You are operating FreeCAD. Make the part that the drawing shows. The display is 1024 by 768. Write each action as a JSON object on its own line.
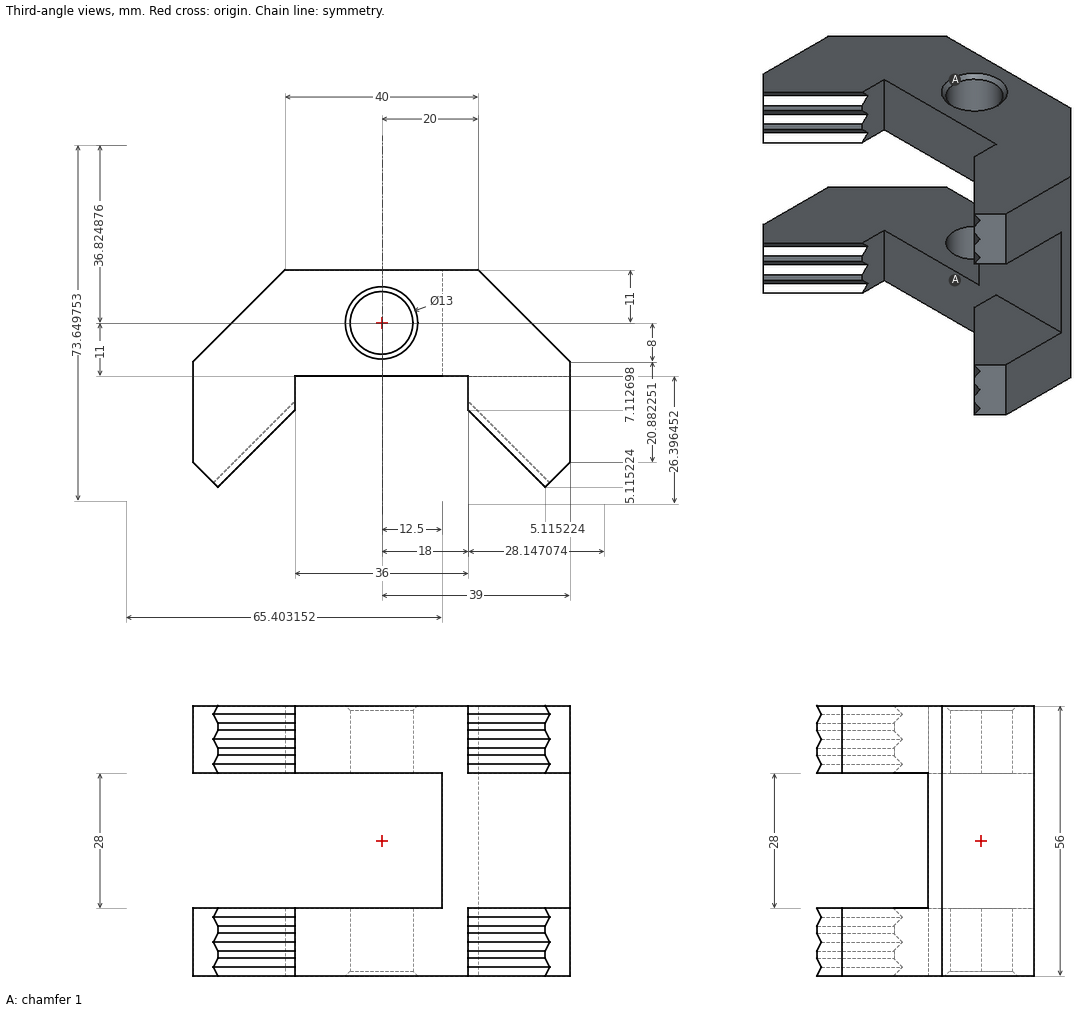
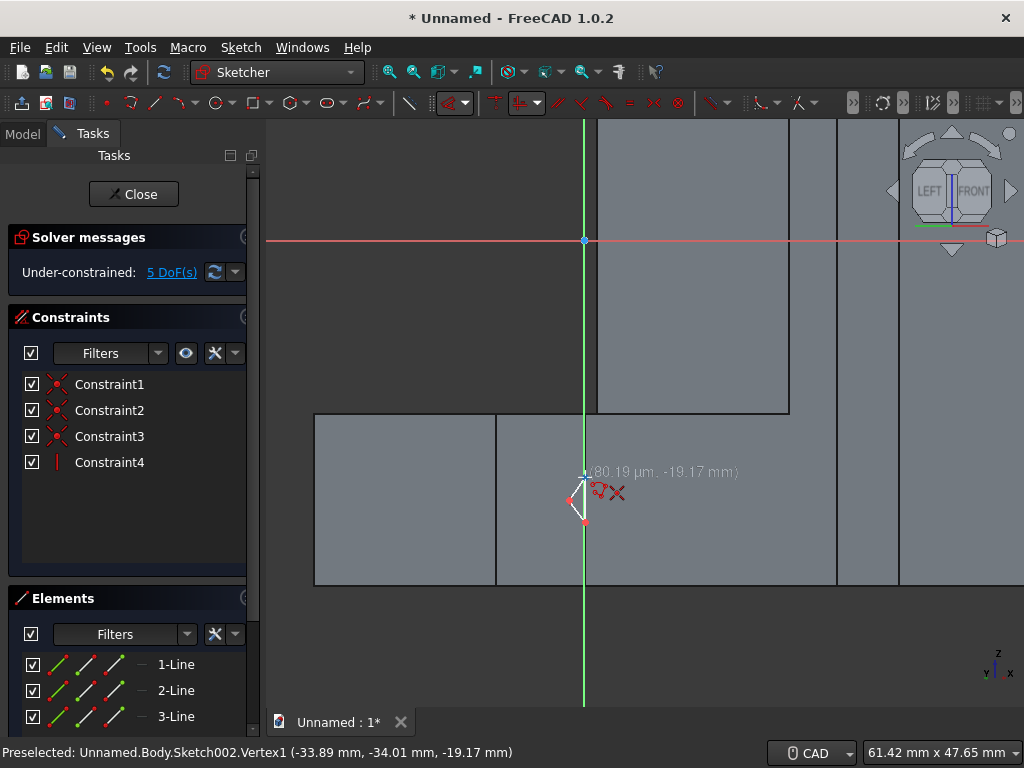
{"action": "scroll", "coordinate": [585, 414], "scroll_direction": "up", "scroll_amount": 14}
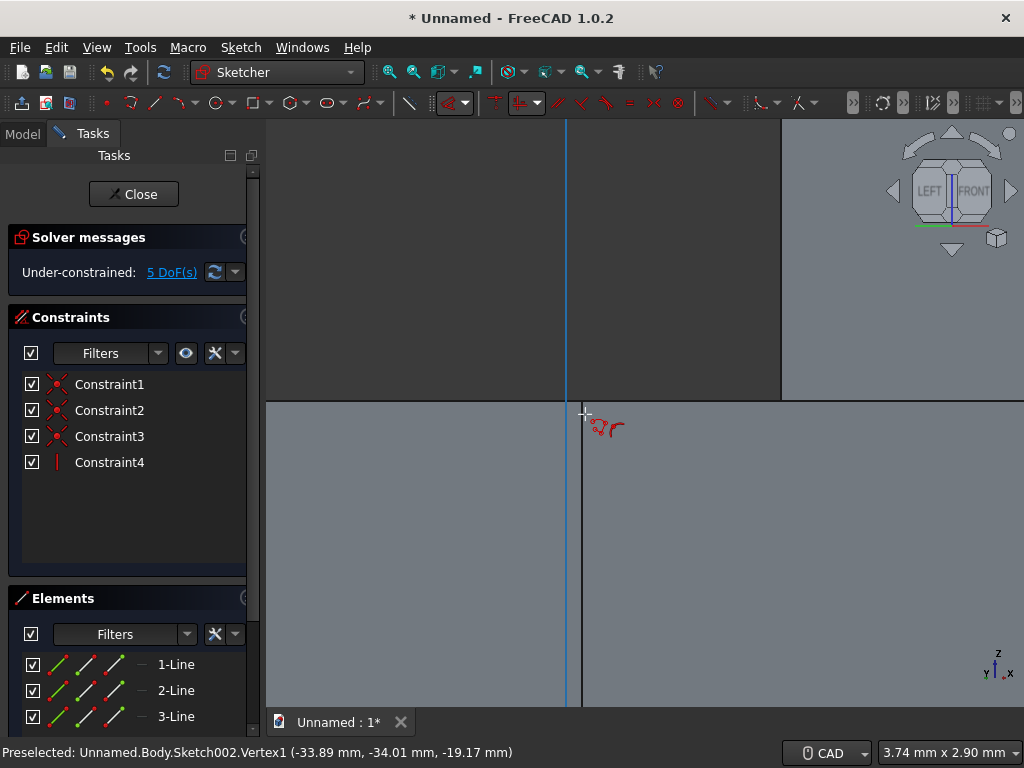
{"action": "left_click", "coordinate": [582, 401]}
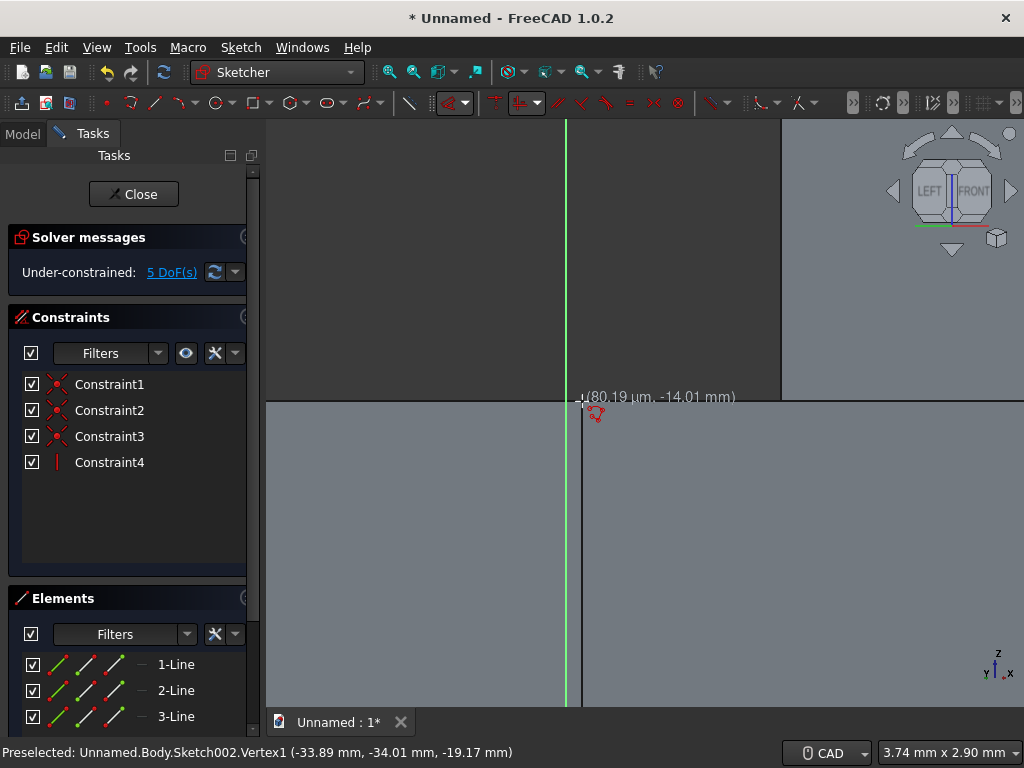
{"action": "scroll", "coordinate": [585, 414], "scroll_direction": "down", "scroll_amount": 14}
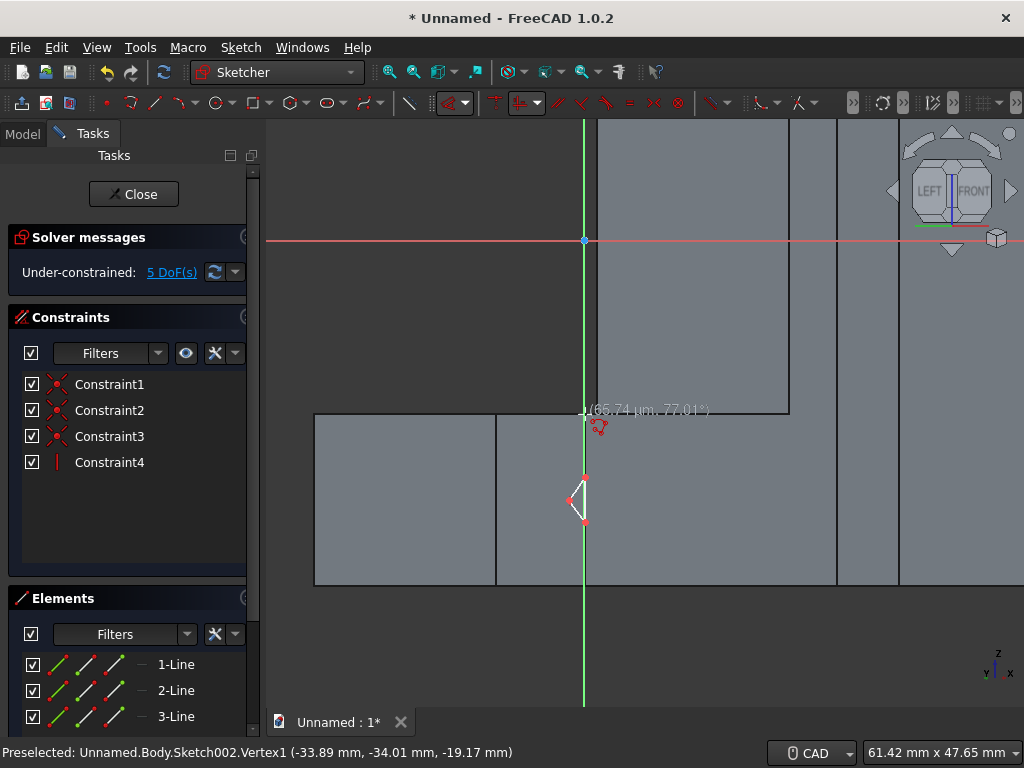
{"action": "left_click", "coordinate": [569, 436]}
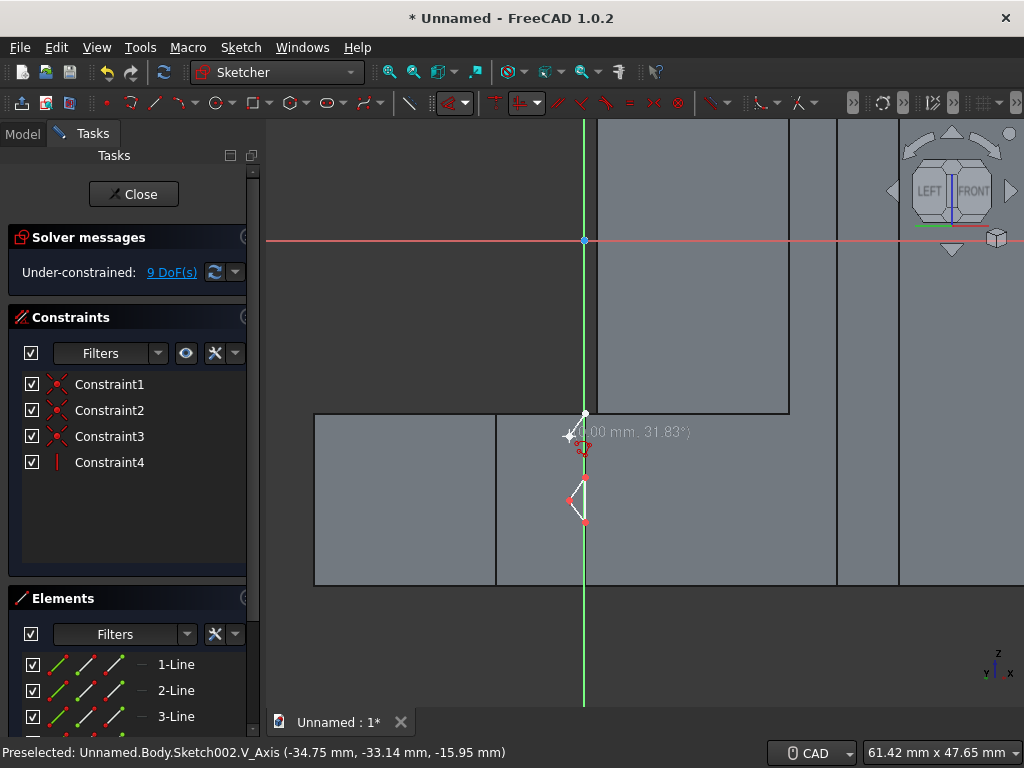
{"action": "scroll", "coordinate": [585, 459], "scroll_direction": "up", "scroll_amount": 14}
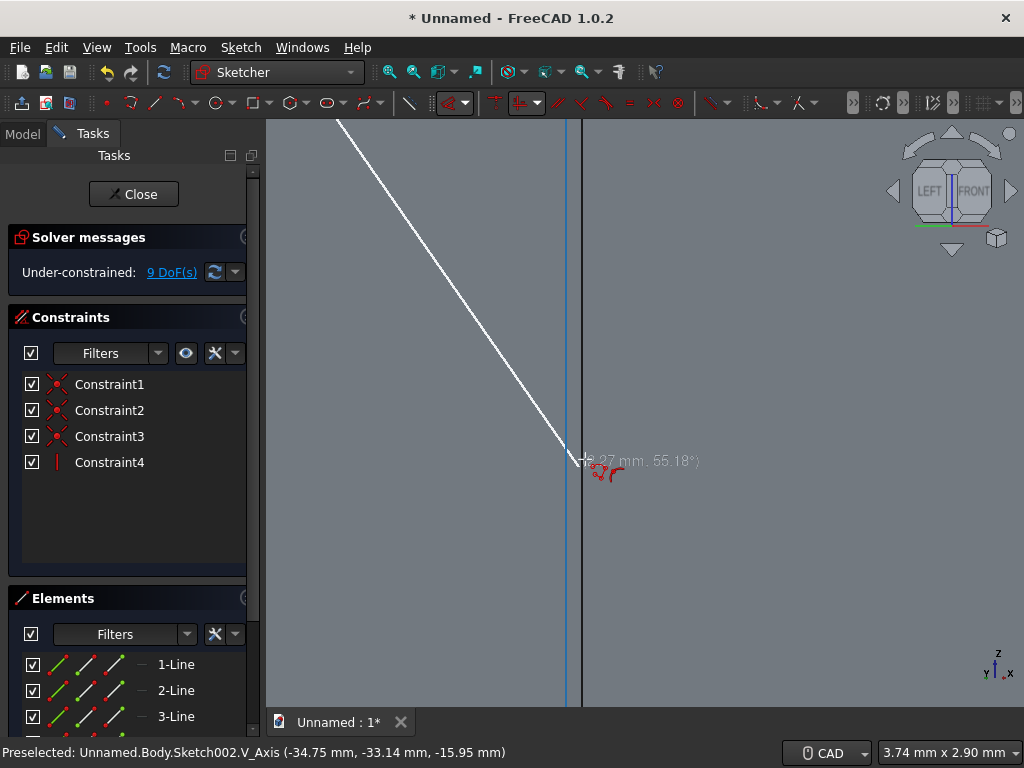
{"action": "left_click", "coordinate": [582, 449]}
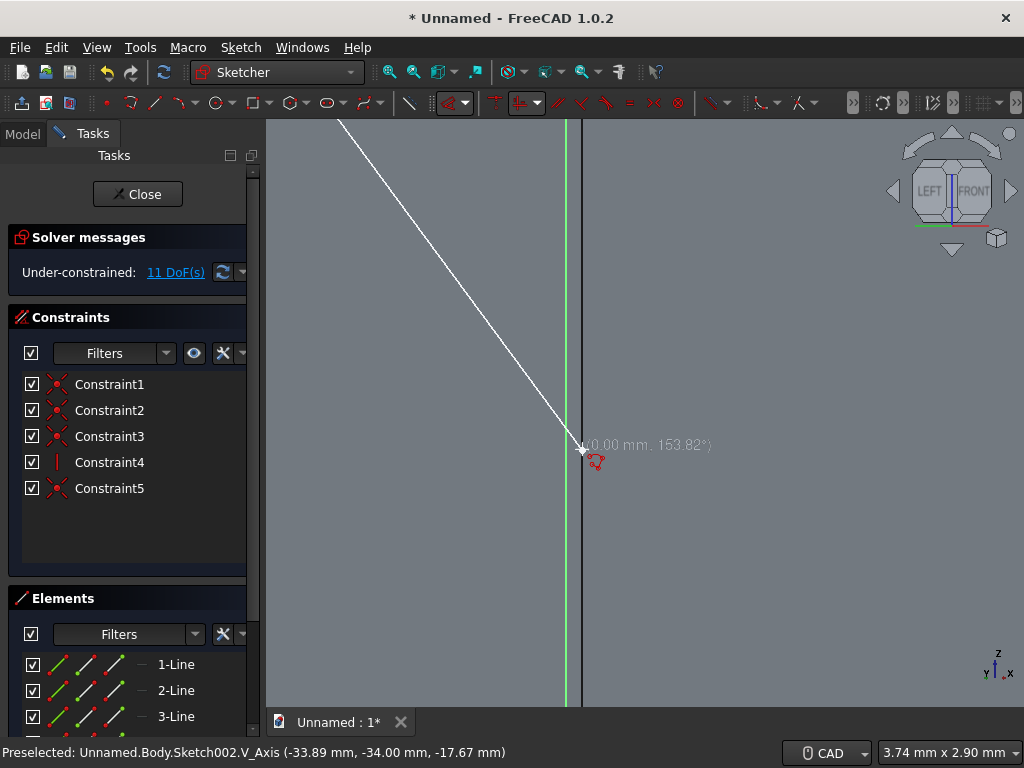
{"action": "scroll", "coordinate": [585, 459], "scroll_direction": "down", "scroll_amount": 14}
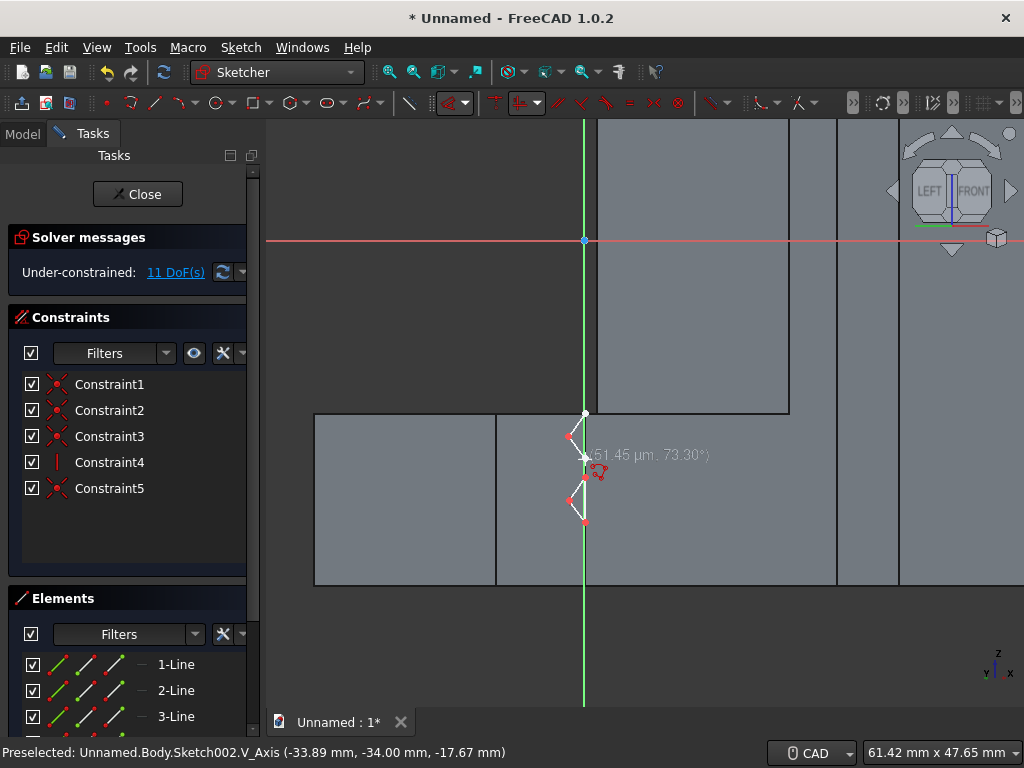
{"action": "scroll", "coordinate": [585, 414], "scroll_direction": "up", "scroll_amount": 14}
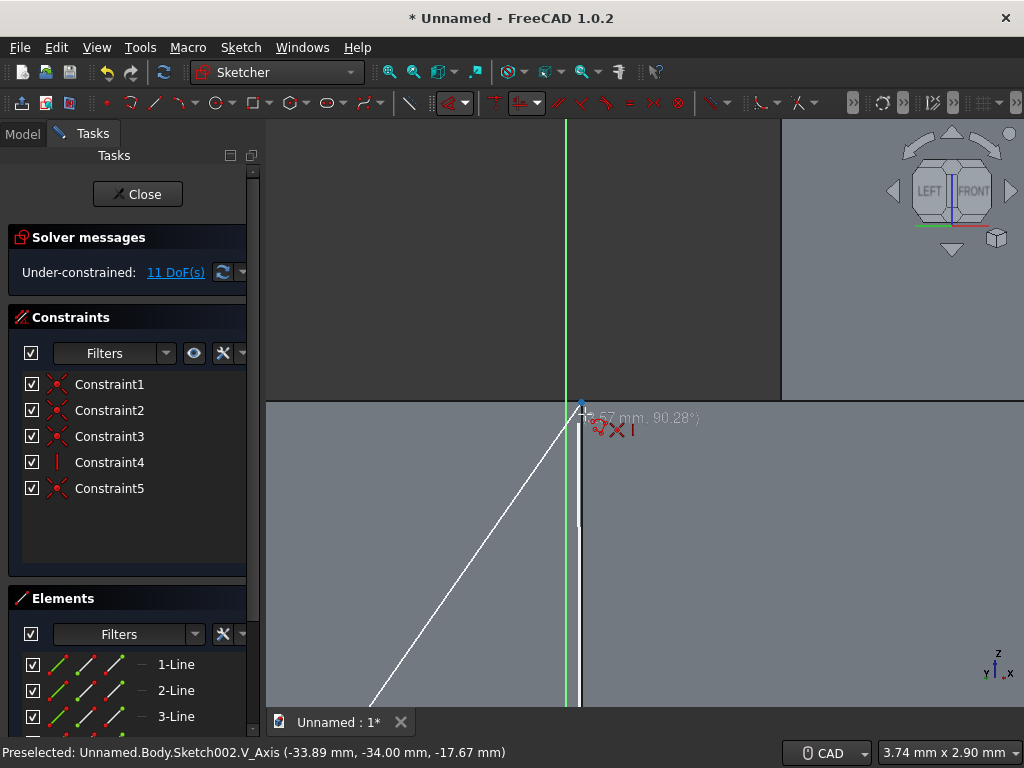
{"action": "left_click", "coordinate": [582, 402]}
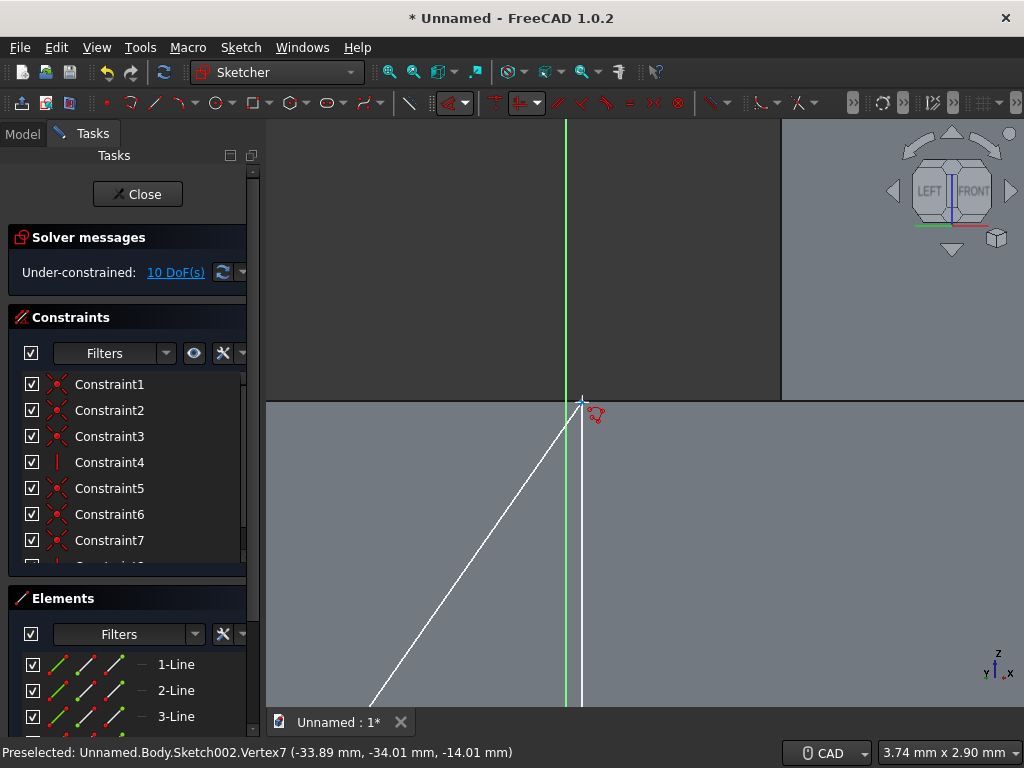
{"action": "scroll", "coordinate": [585, 414], "scroll_direction": "down", "scroll_amount": 14}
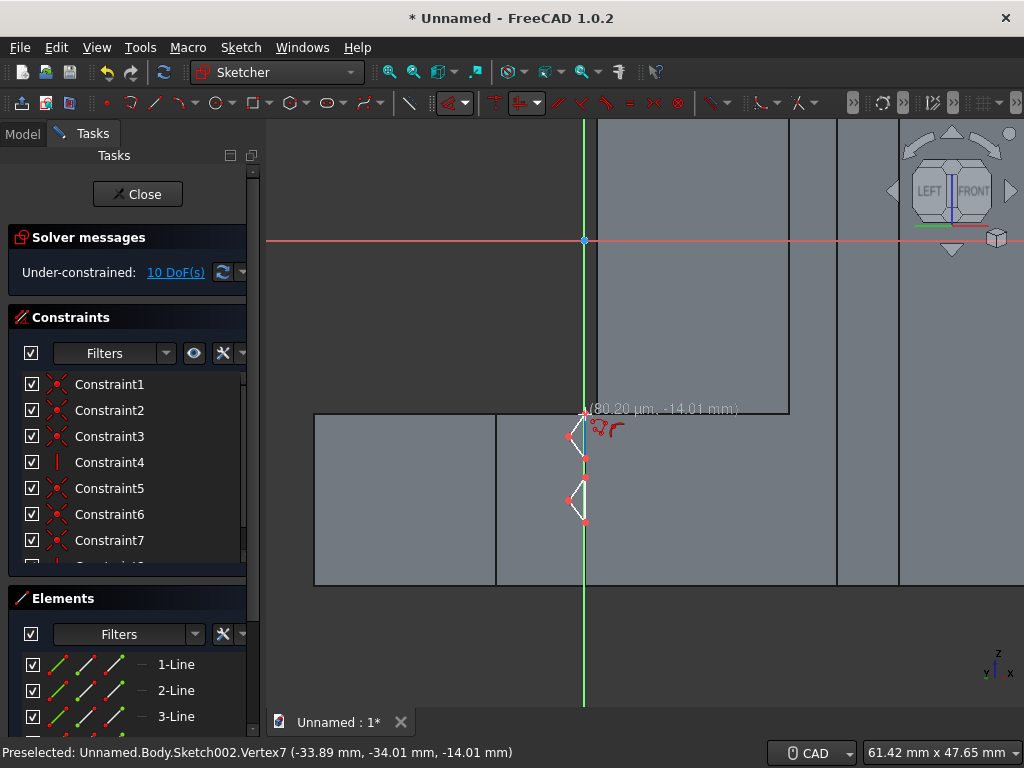
{"action": "scroll", "coordinate": [585, 541], "scroll_direction": "up", "scroll_amount": 14}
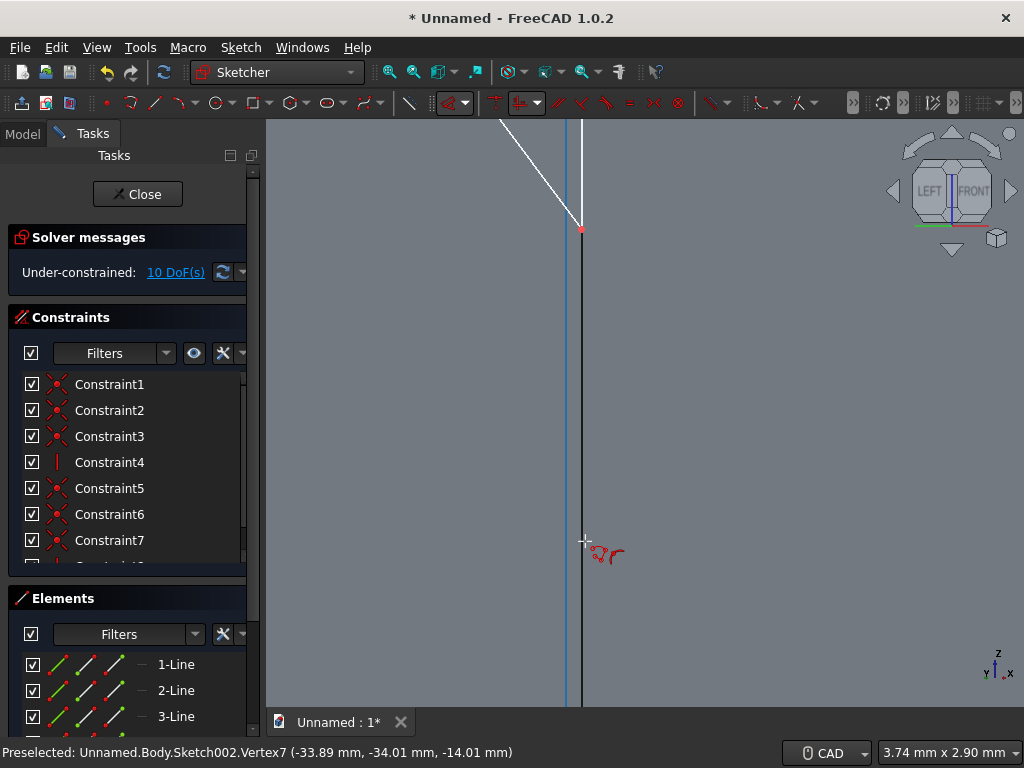
{"action": "left_click", "coordinate": [582, 533]}